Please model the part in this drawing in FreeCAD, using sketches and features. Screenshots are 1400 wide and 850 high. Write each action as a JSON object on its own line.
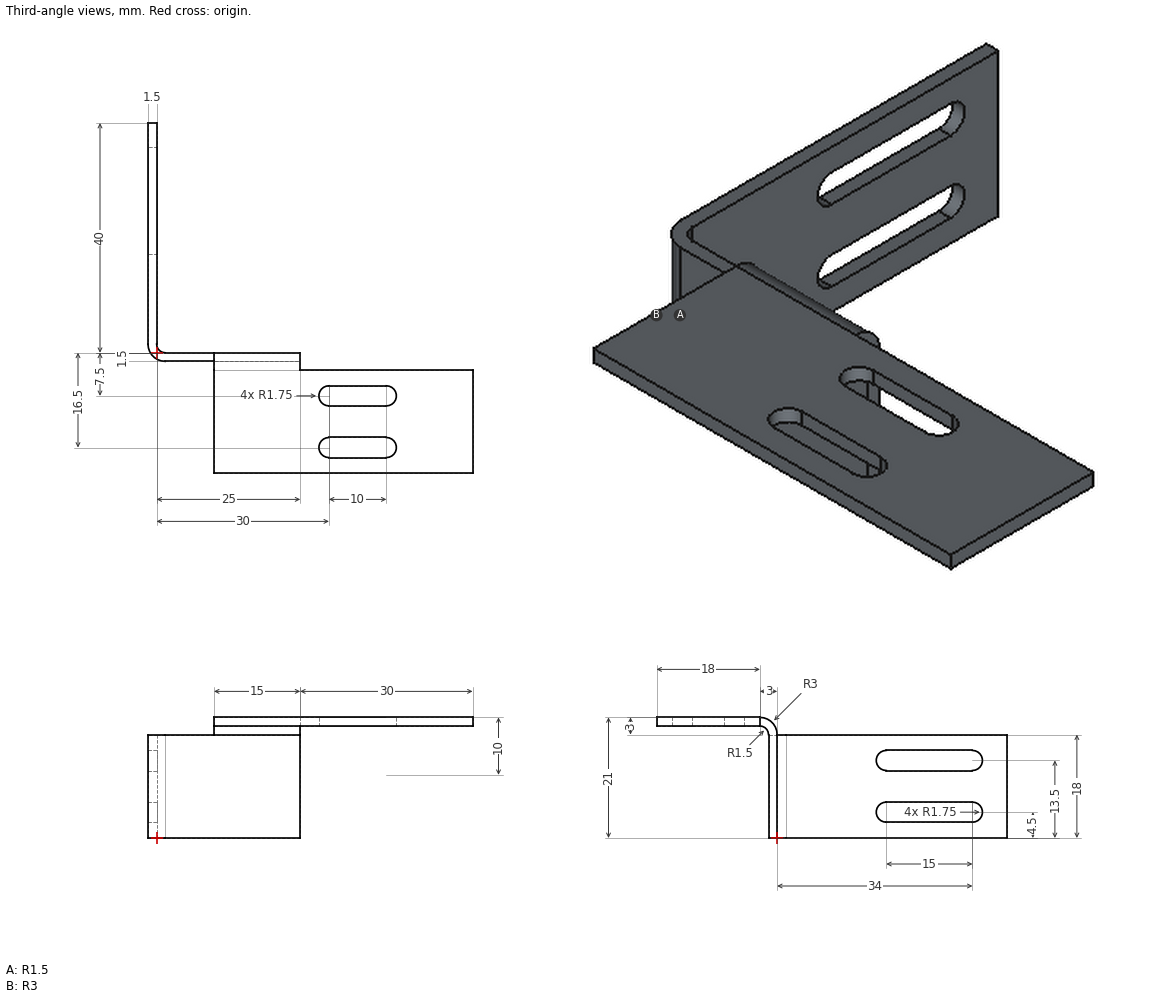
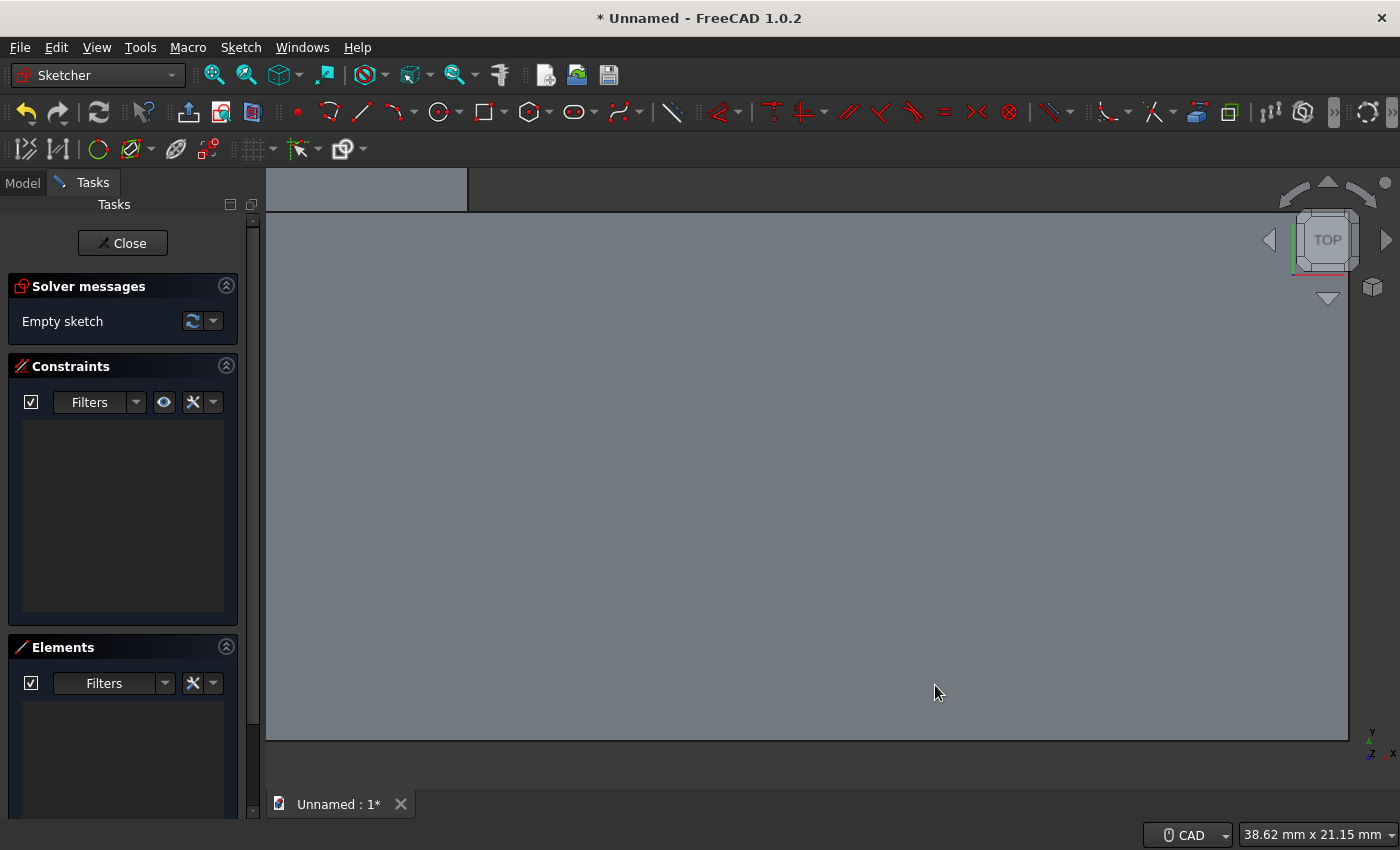
{"action": "key", "text": "g s"}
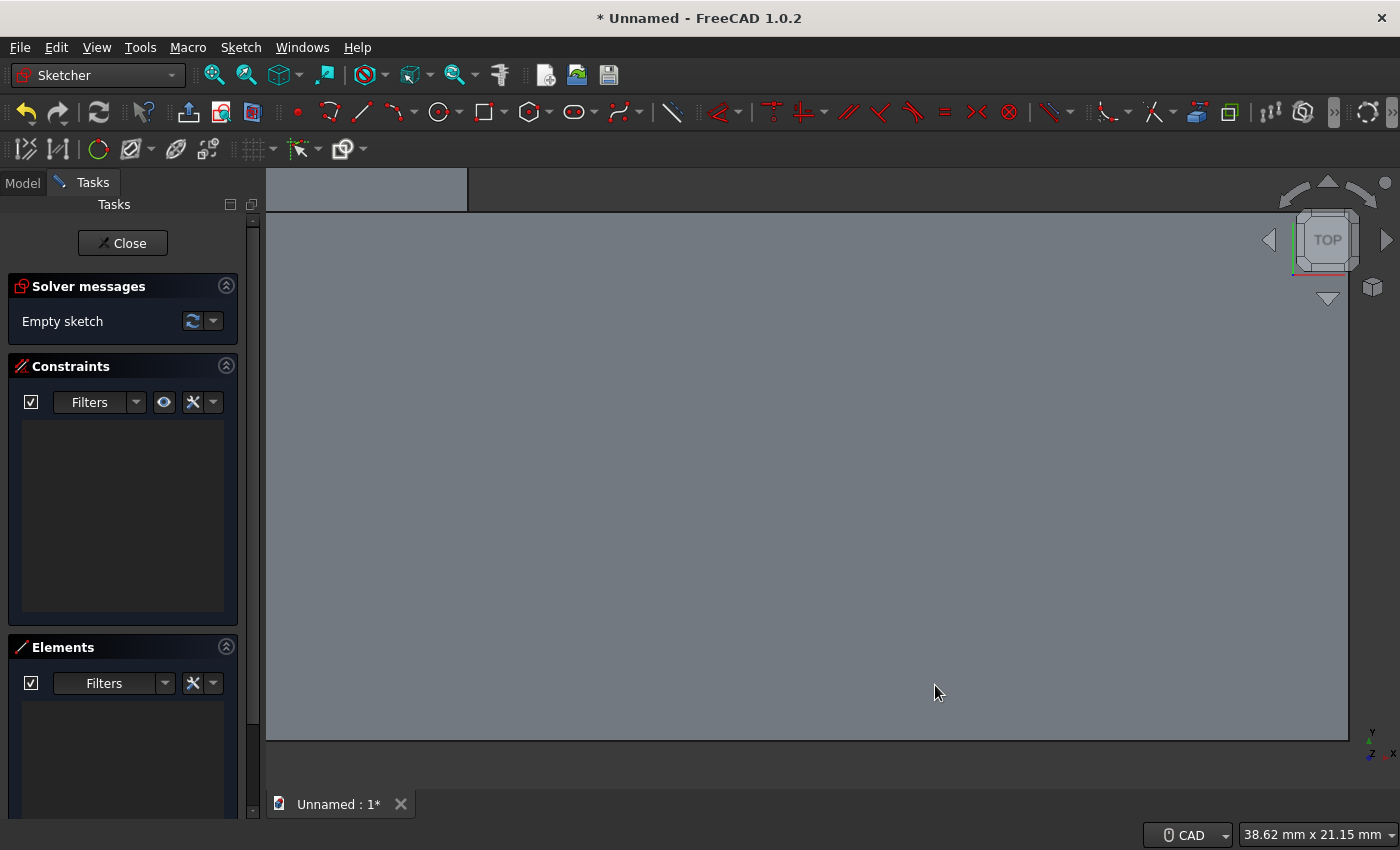
{"action": "left_click", "coordinate": [615, 344]}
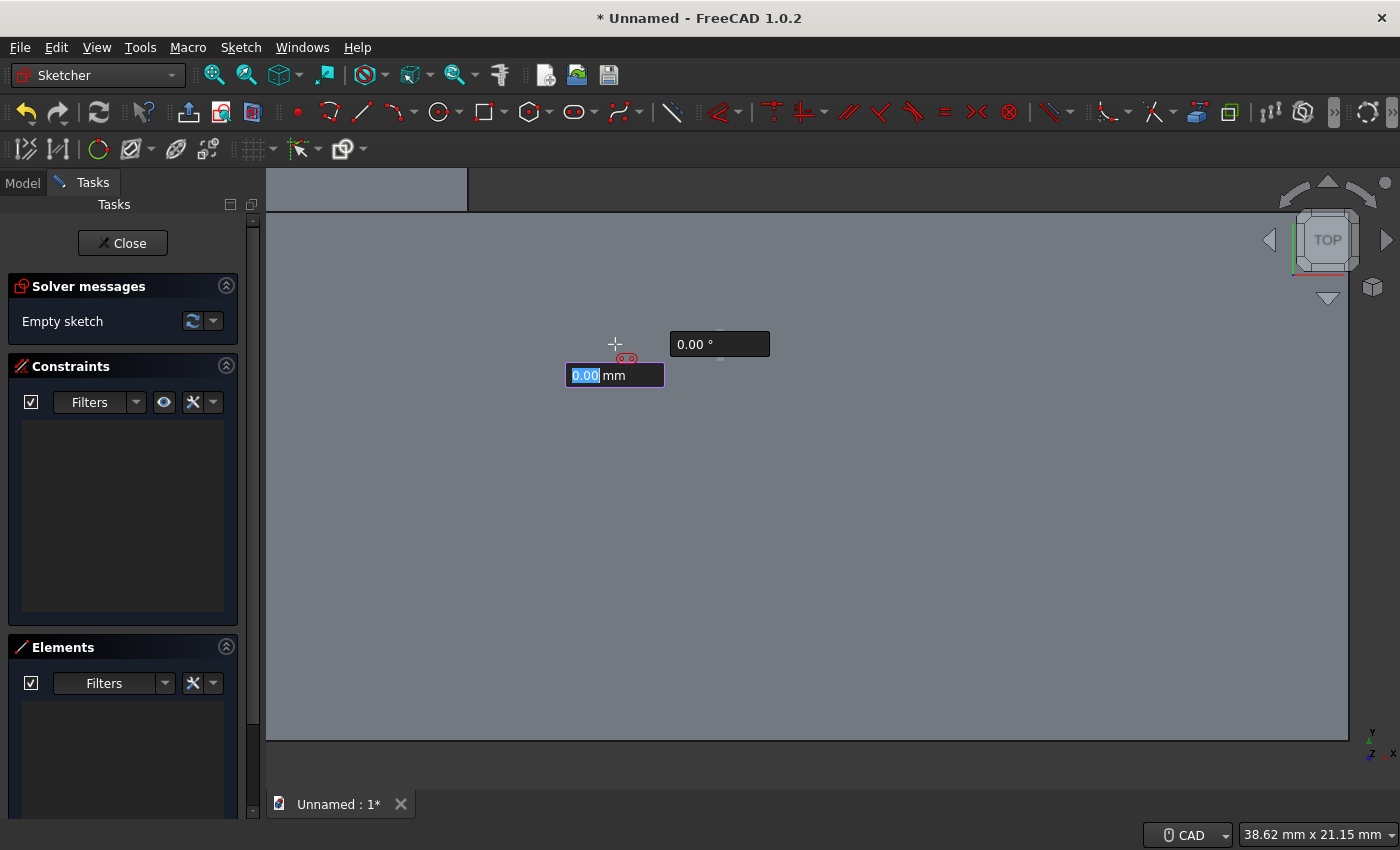
{"action": "left_click", "coordinate": [909, 344]}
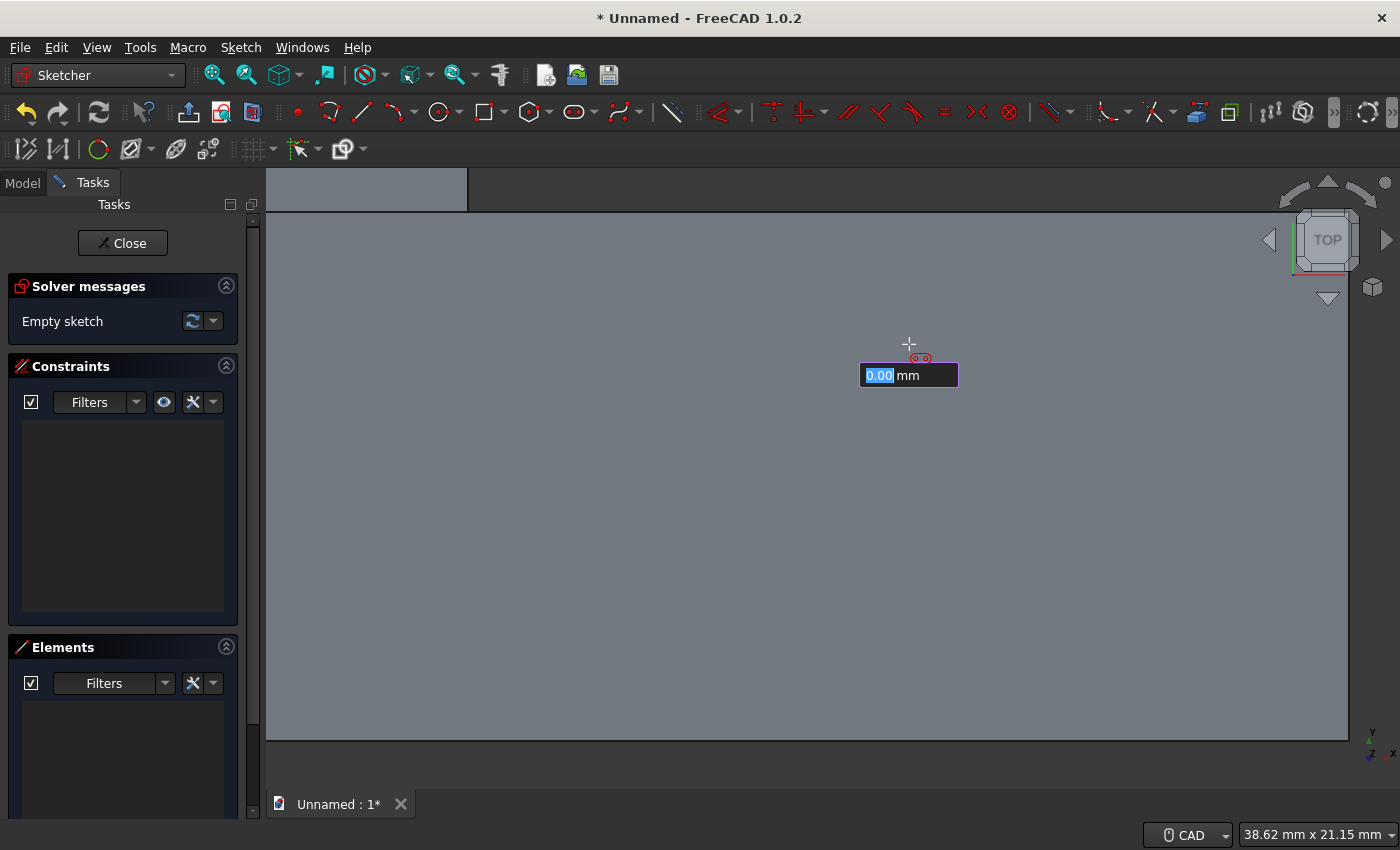
{"action": "left_click", "coordinate": [762, 293]}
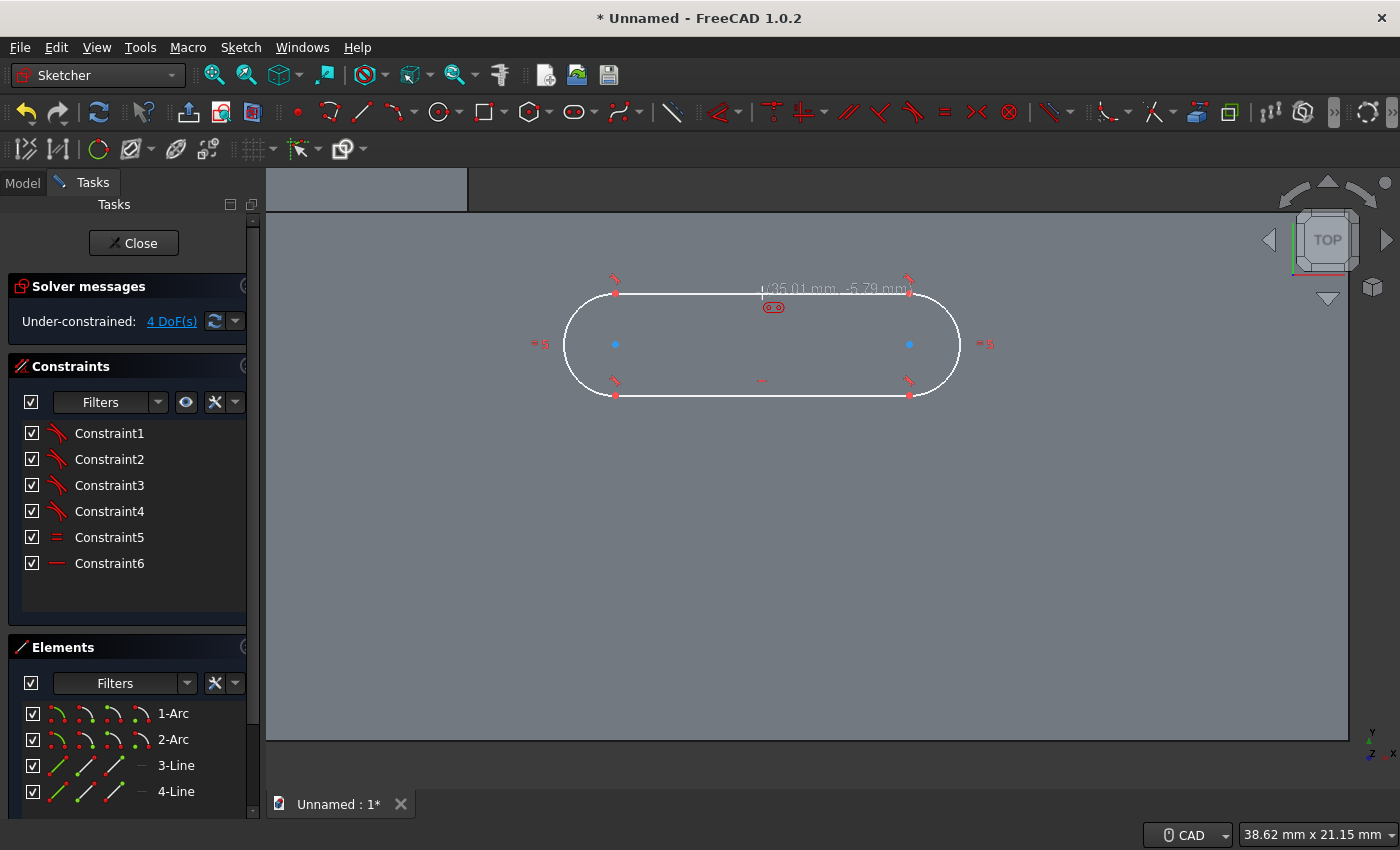
{"action": "left_click", "coordinate": [615, 609]}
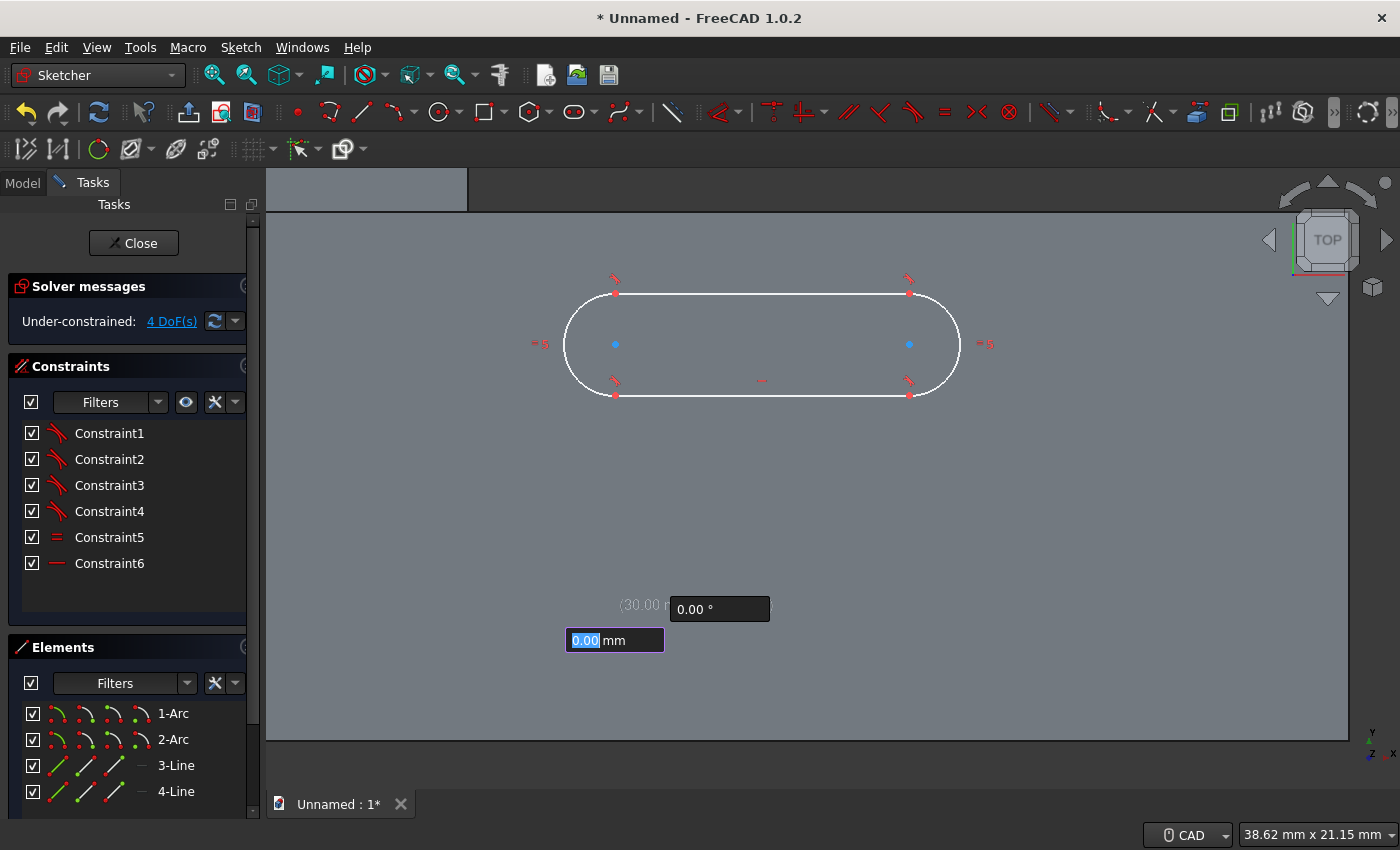
{"action": "left_click", "coordinate": [909, 609]}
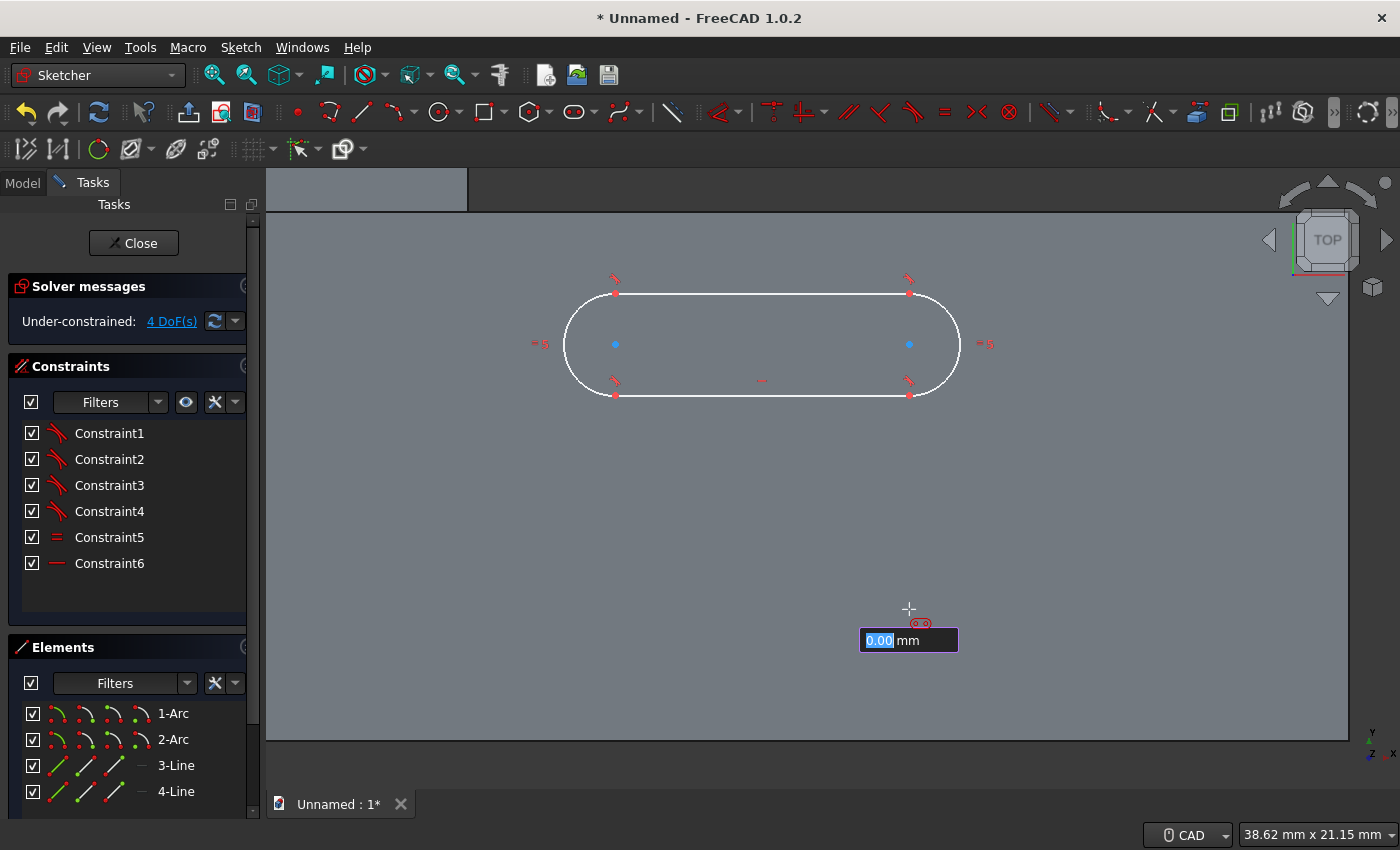
{"action": "left_click", "coordinate": [762, 660]}
{"action": "key", "text": "Escape"}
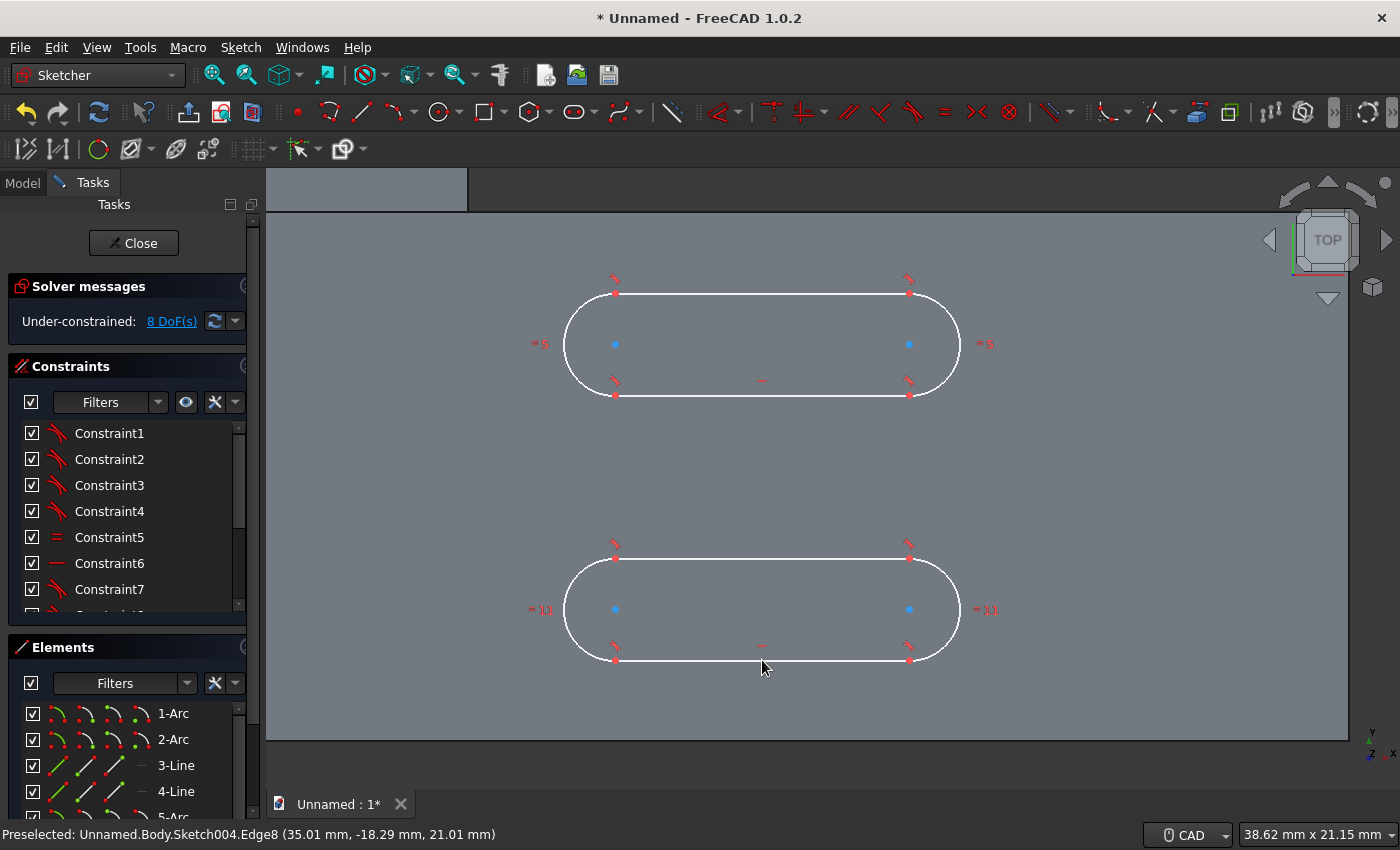
{"action": "left_click", "coordinate": [574, 315]}